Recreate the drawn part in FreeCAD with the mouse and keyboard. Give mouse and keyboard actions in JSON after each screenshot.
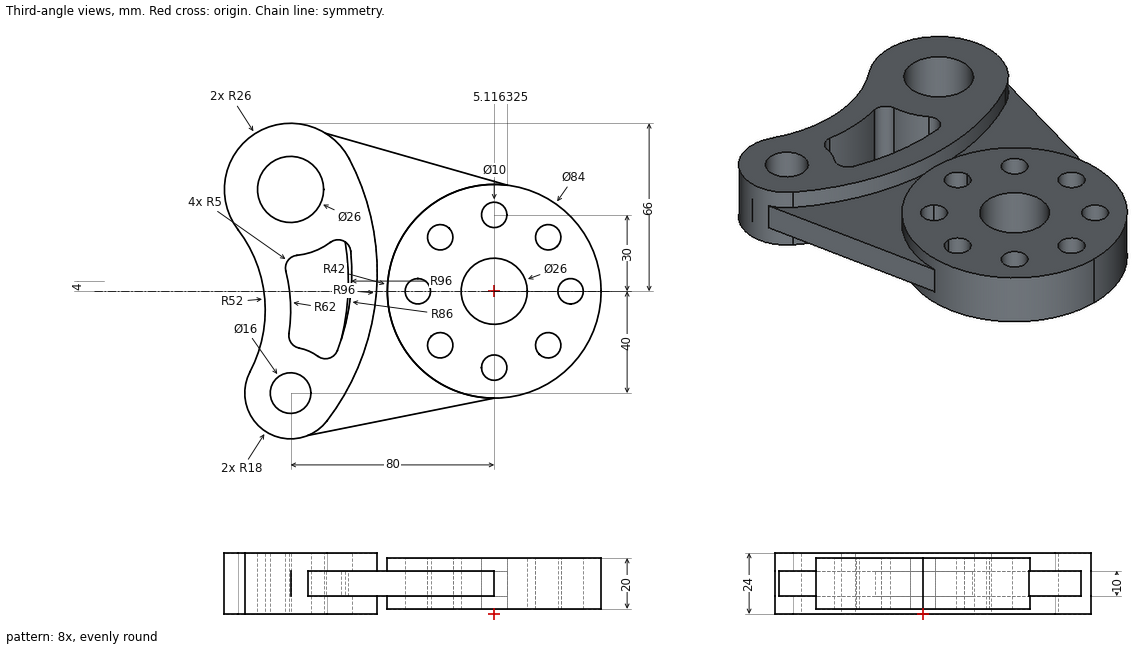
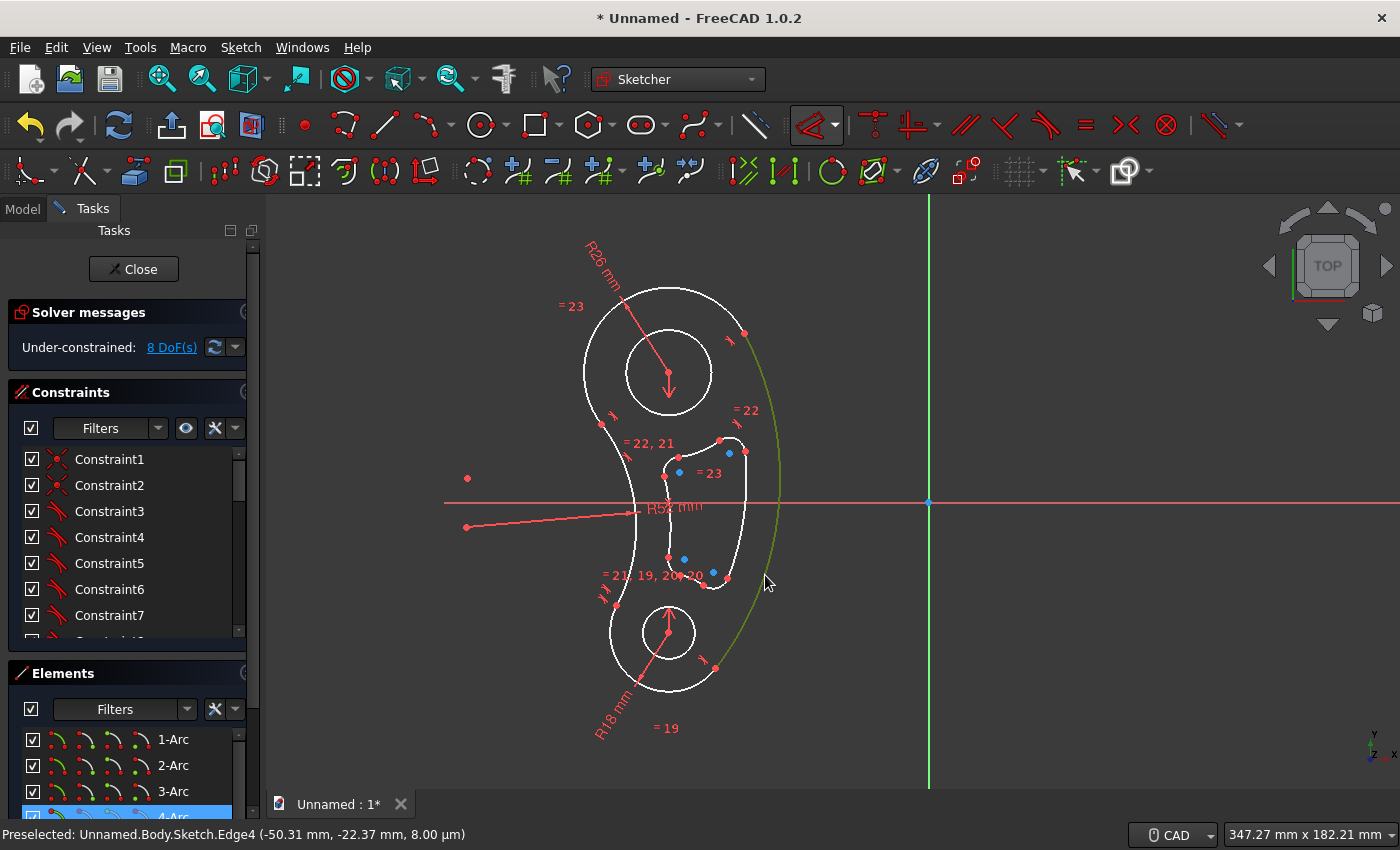
{"action": "left_click", "coordinate": [838, 126]}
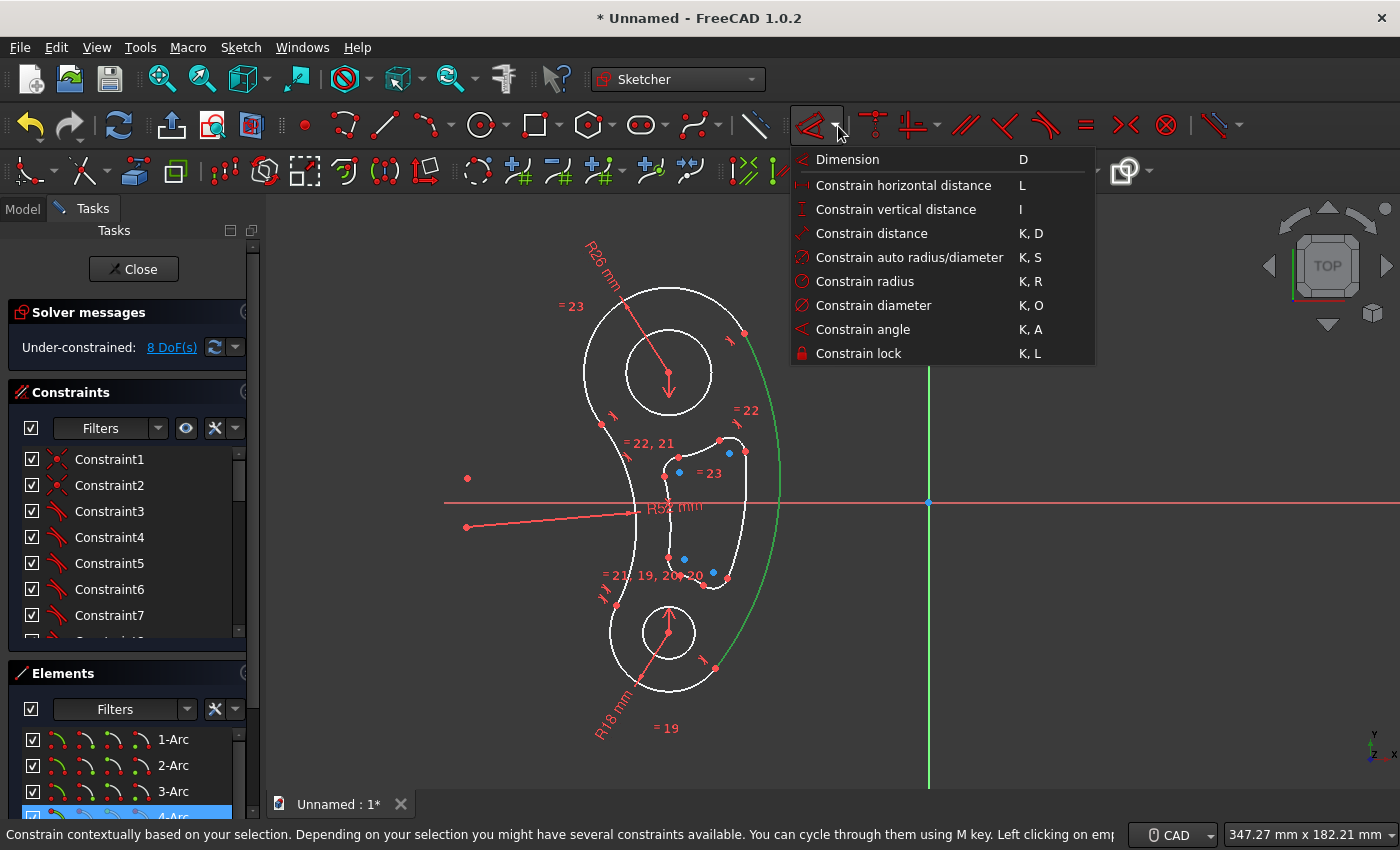
{"action": "left_click", "coordinate": [943, 281]}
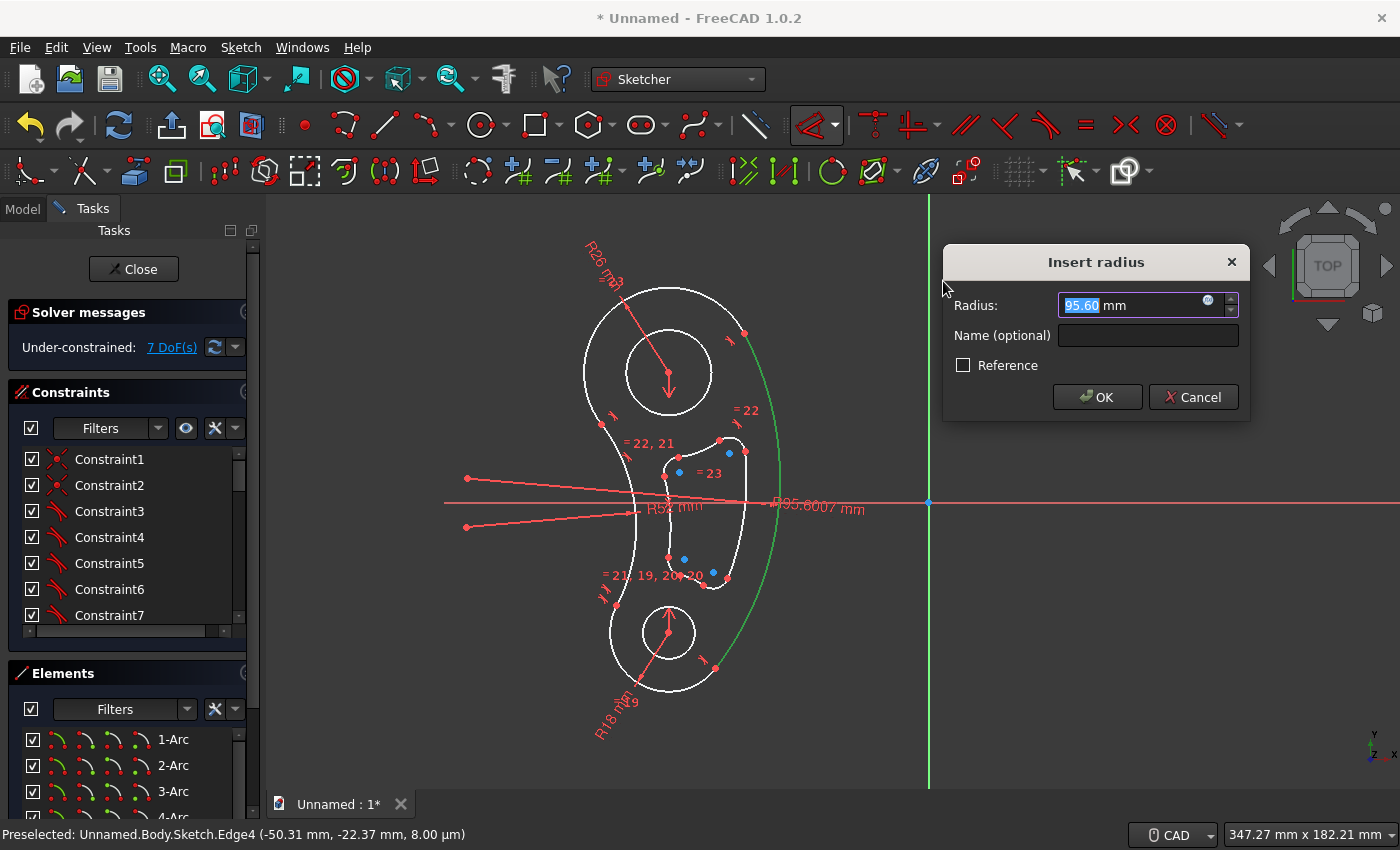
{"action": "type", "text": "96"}
{"action": "key", "text": "Return"}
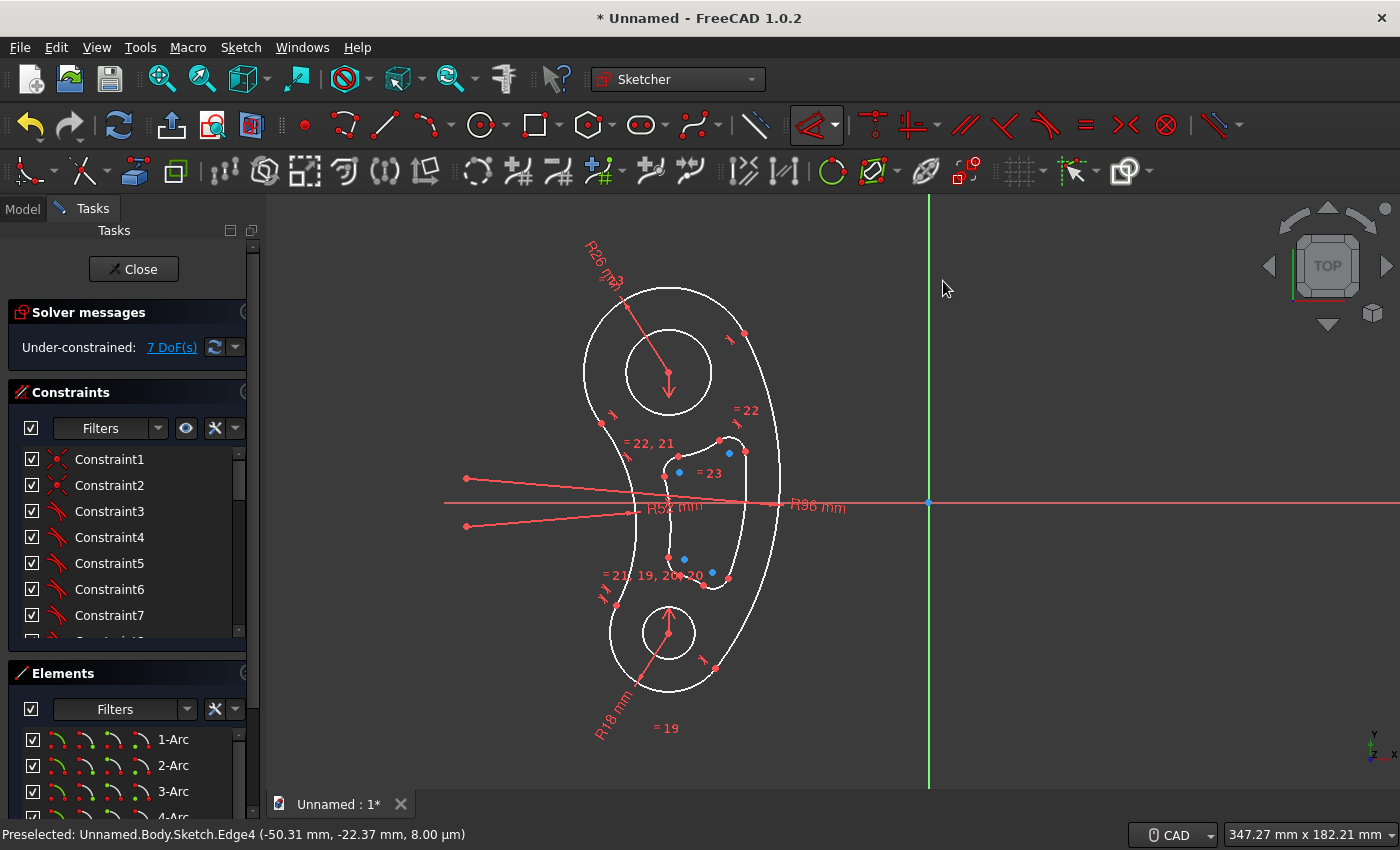
{"action": "left_click", "coordinate": [739, 541]}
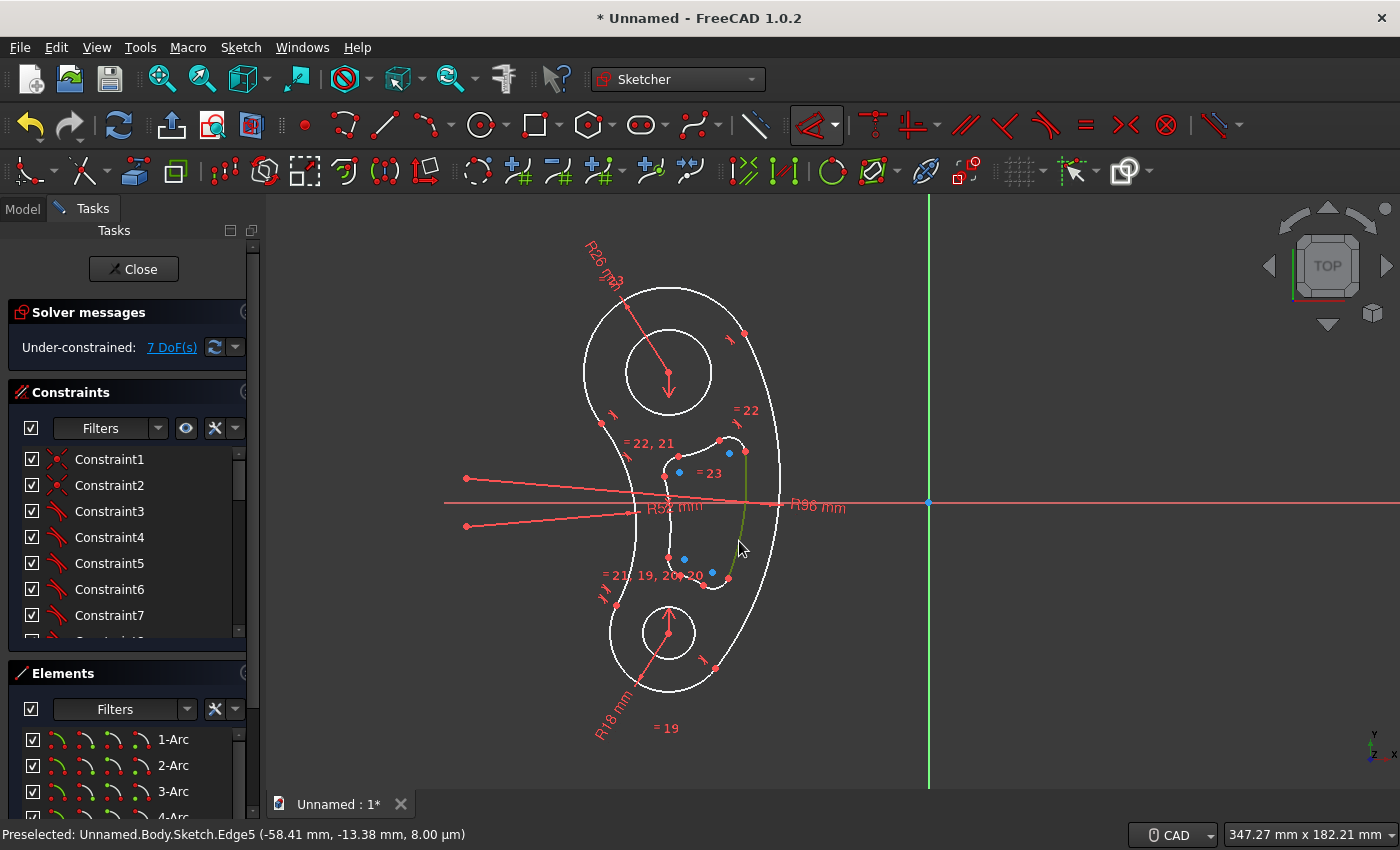
{"action": "key", "text": "k r"}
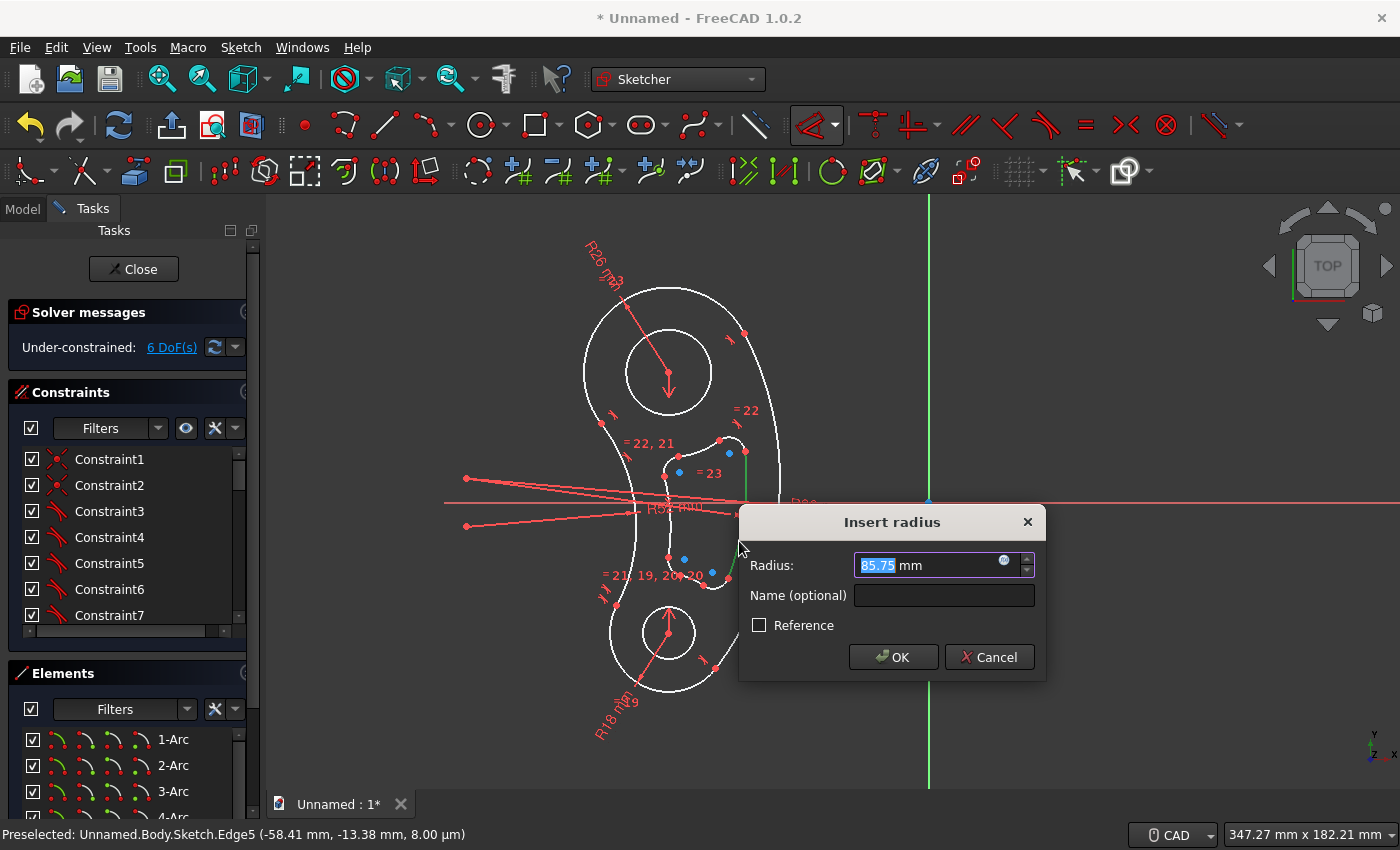
{"action": "type", "text": "86"}
{"action": "key", "text": "Return"}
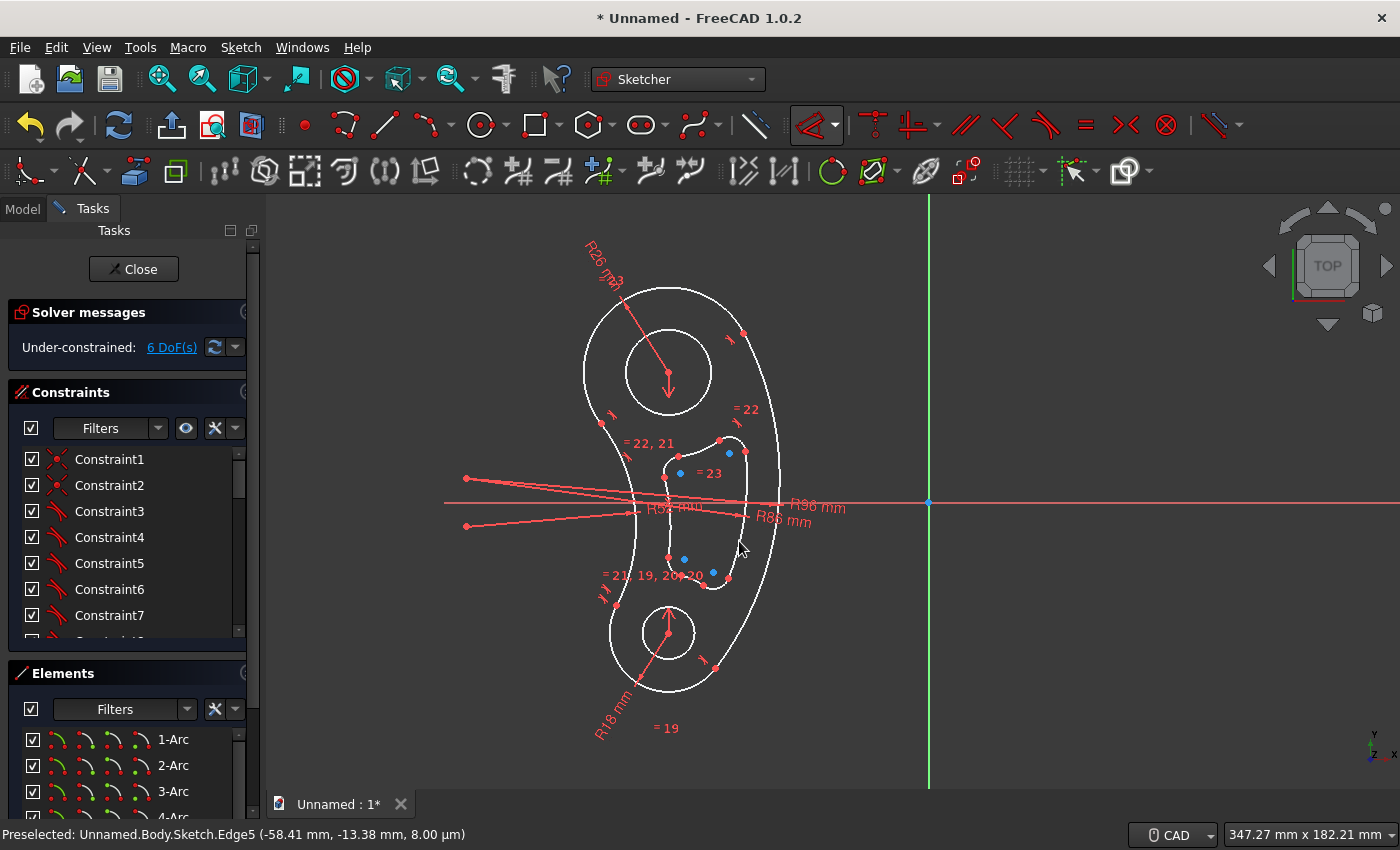
{"action": "scroll", "coordinate": [718, 588], "scroll_direction": "up", "scroll_amount": 5}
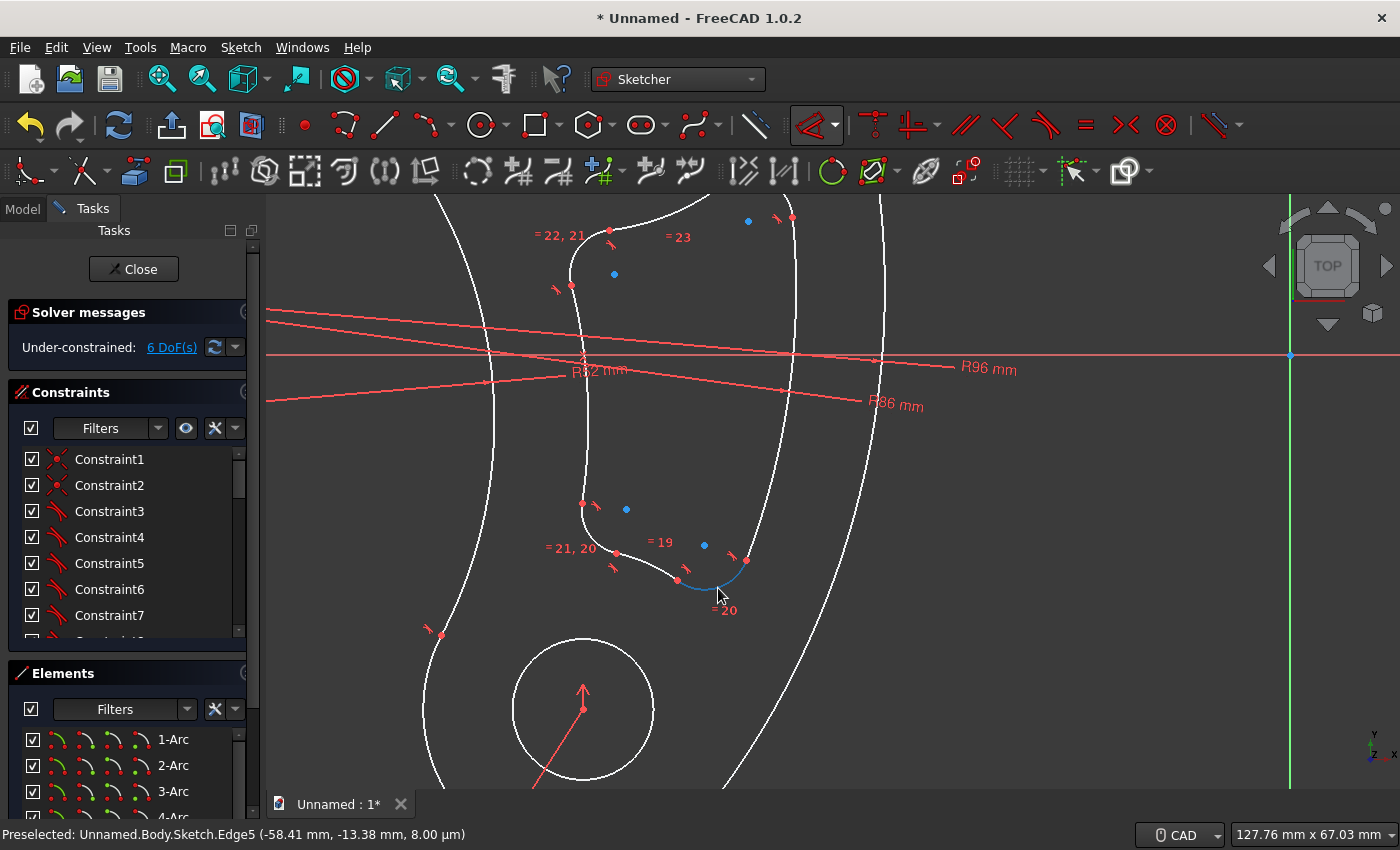
{"action": "left_click", "coordinate": [717, 588]}